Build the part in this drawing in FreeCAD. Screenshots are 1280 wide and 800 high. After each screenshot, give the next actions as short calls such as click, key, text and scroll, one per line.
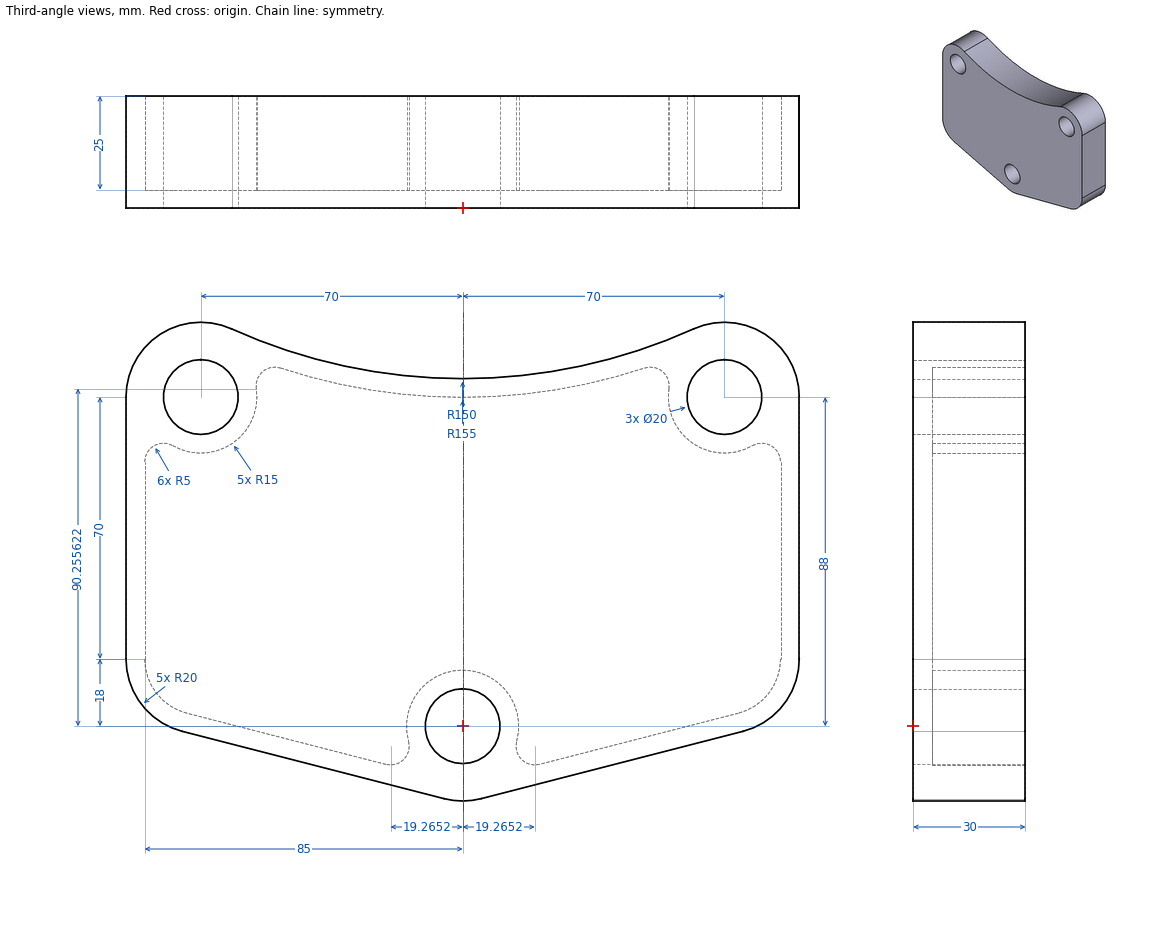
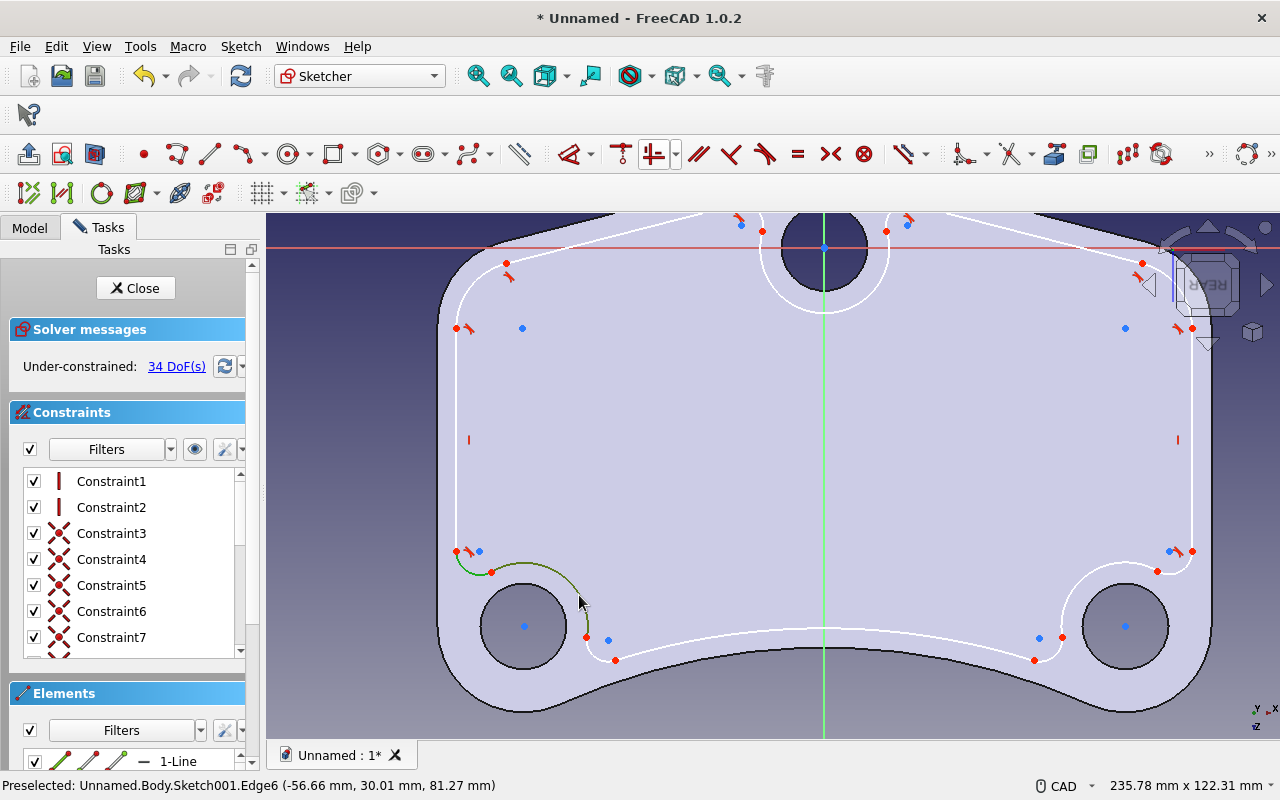
click(765, 154)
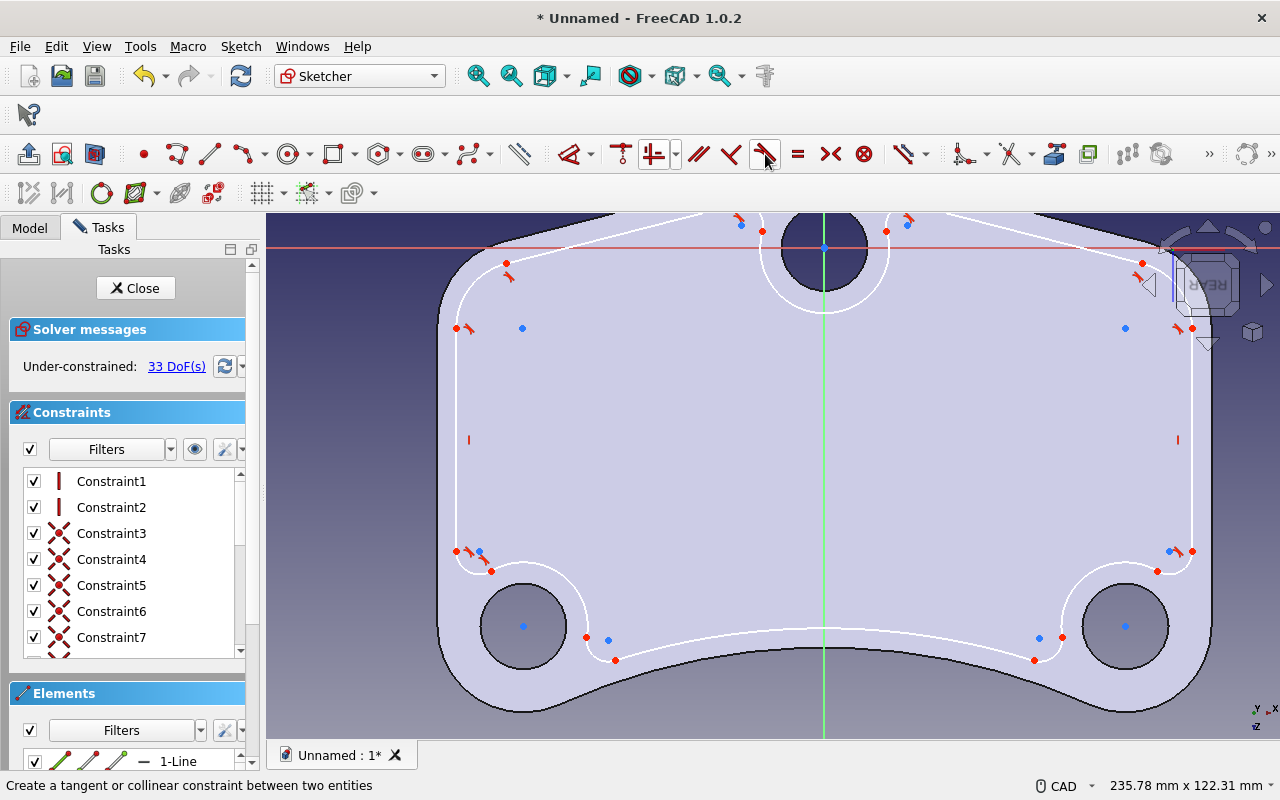
click(579, 595)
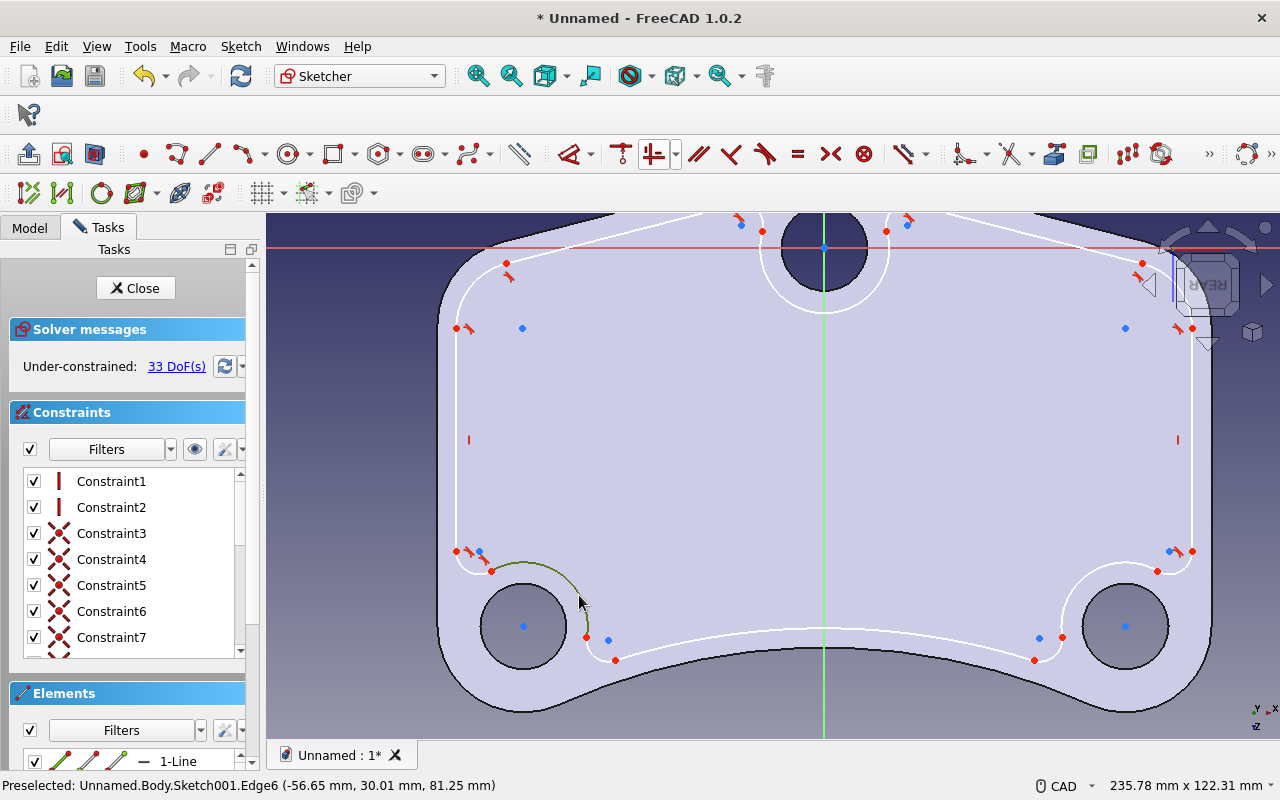
click(589, 650)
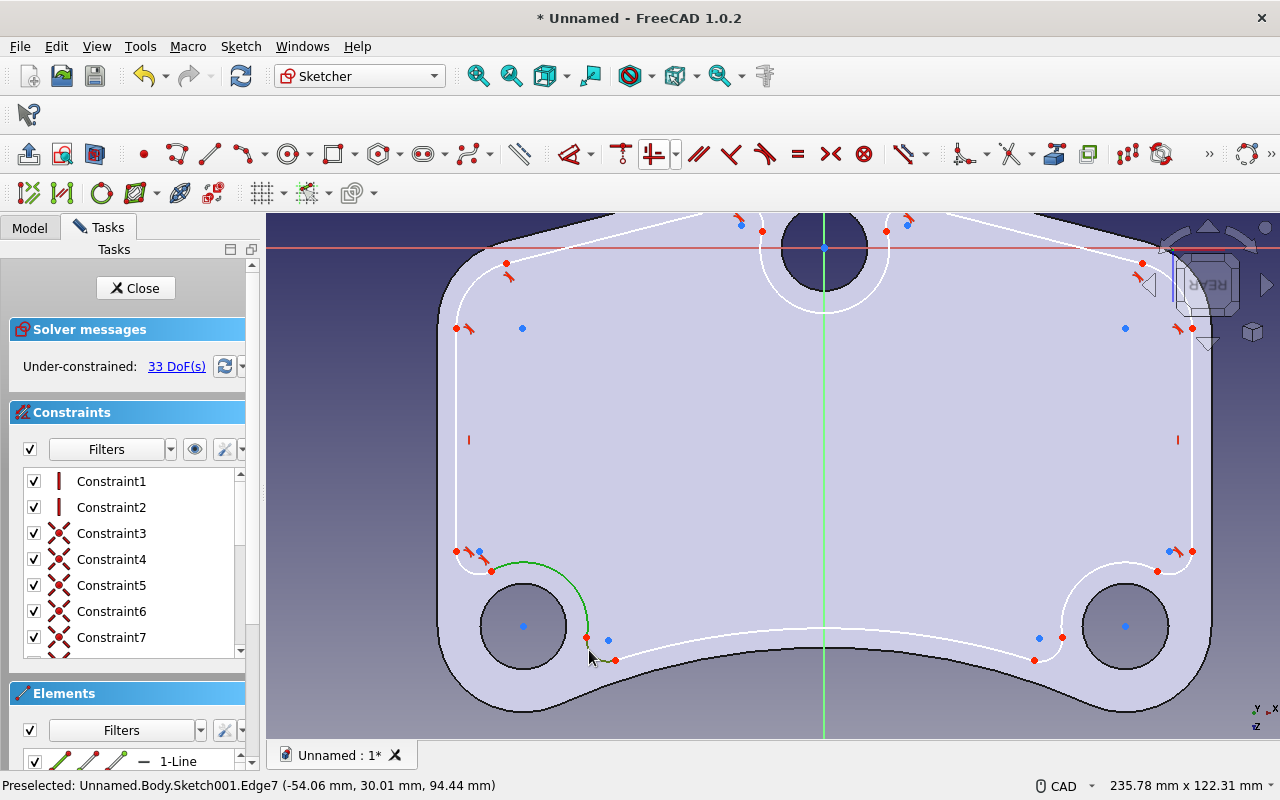
click(765, 154)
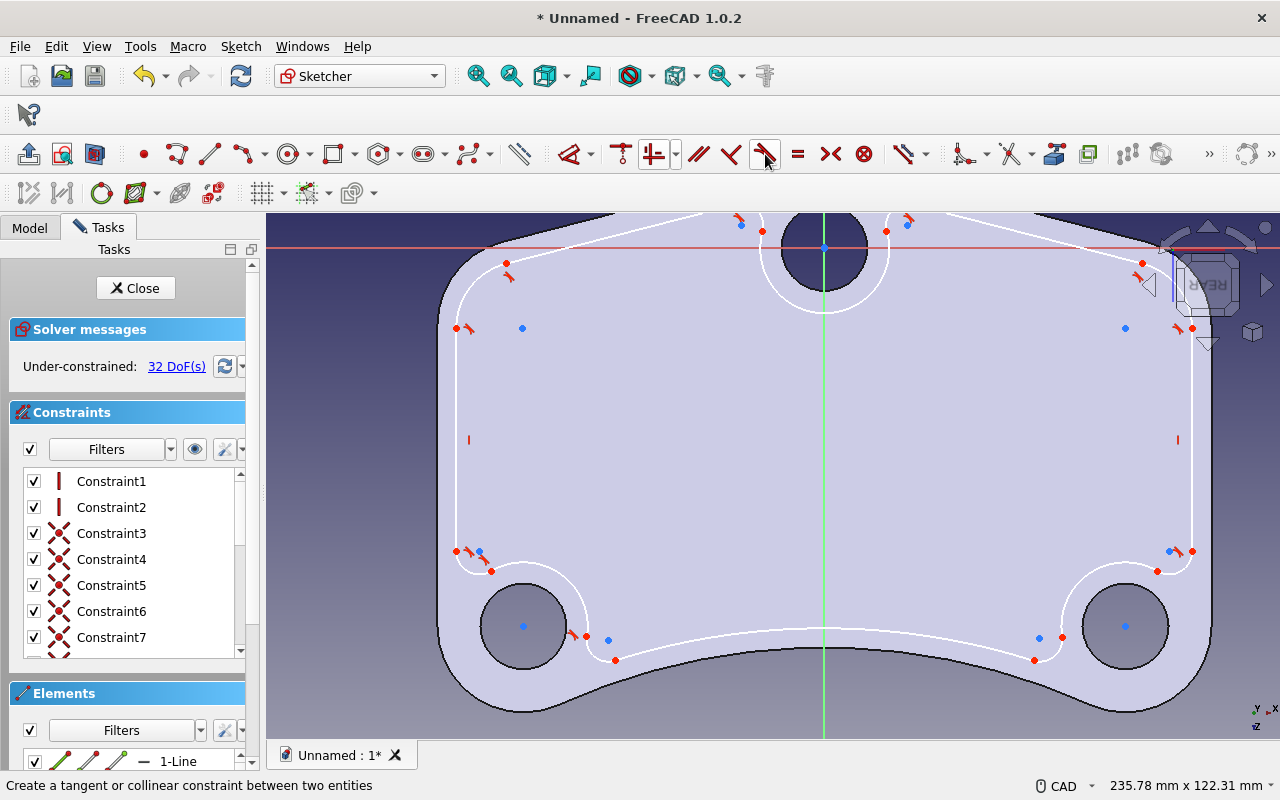
click(589, 650)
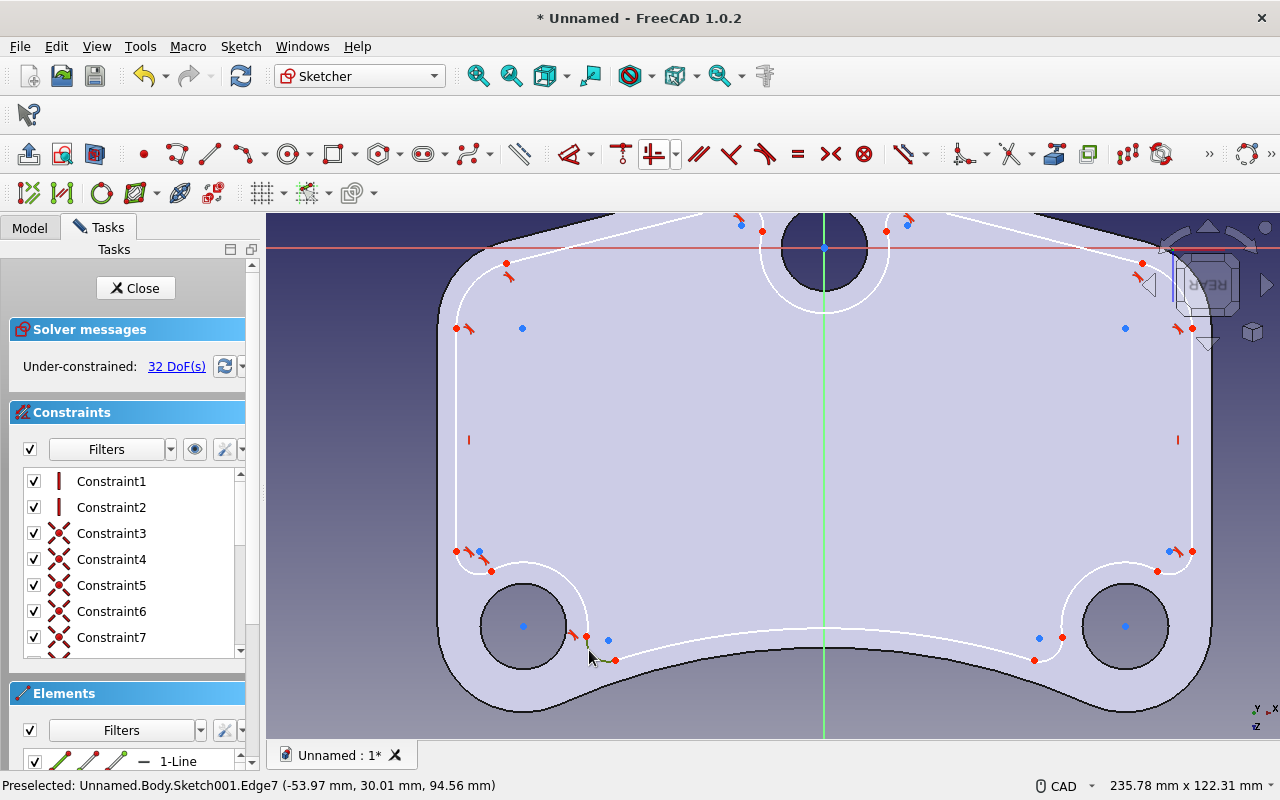
click(909, 634)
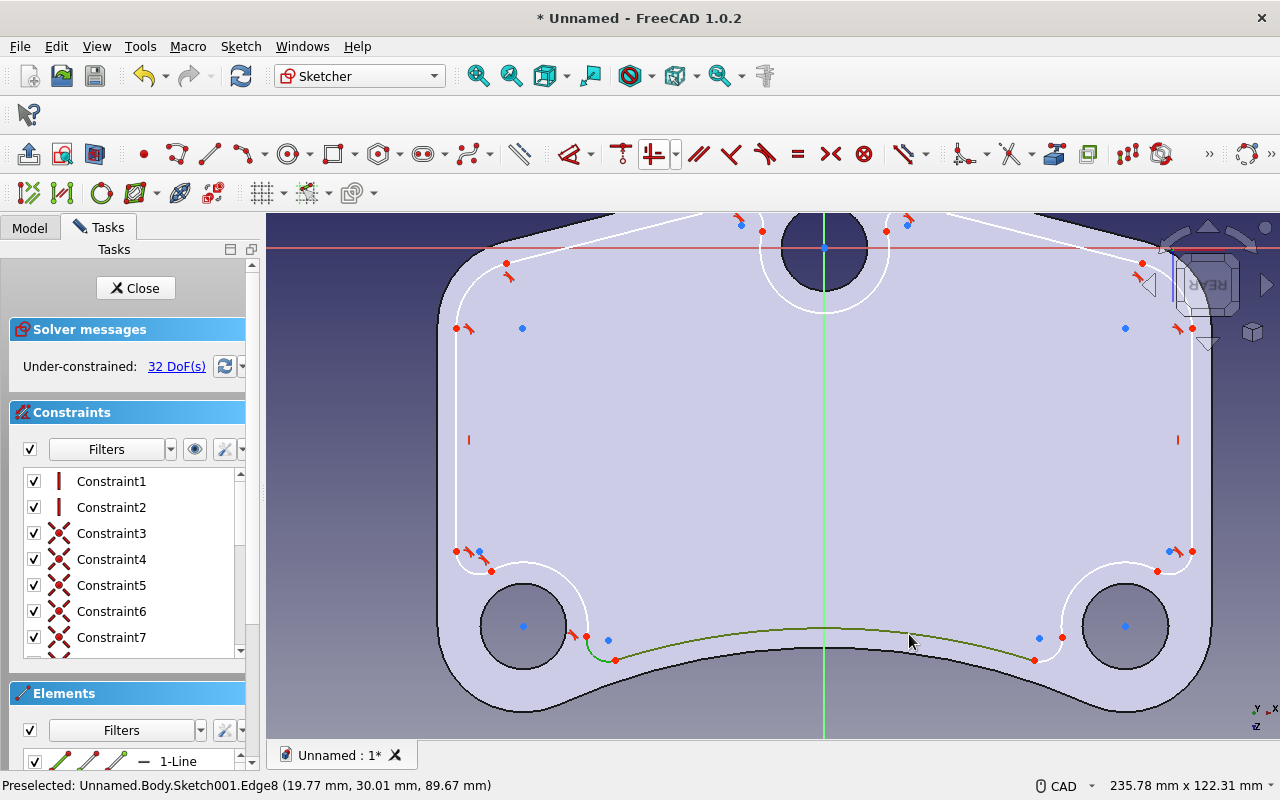
click(765, 154)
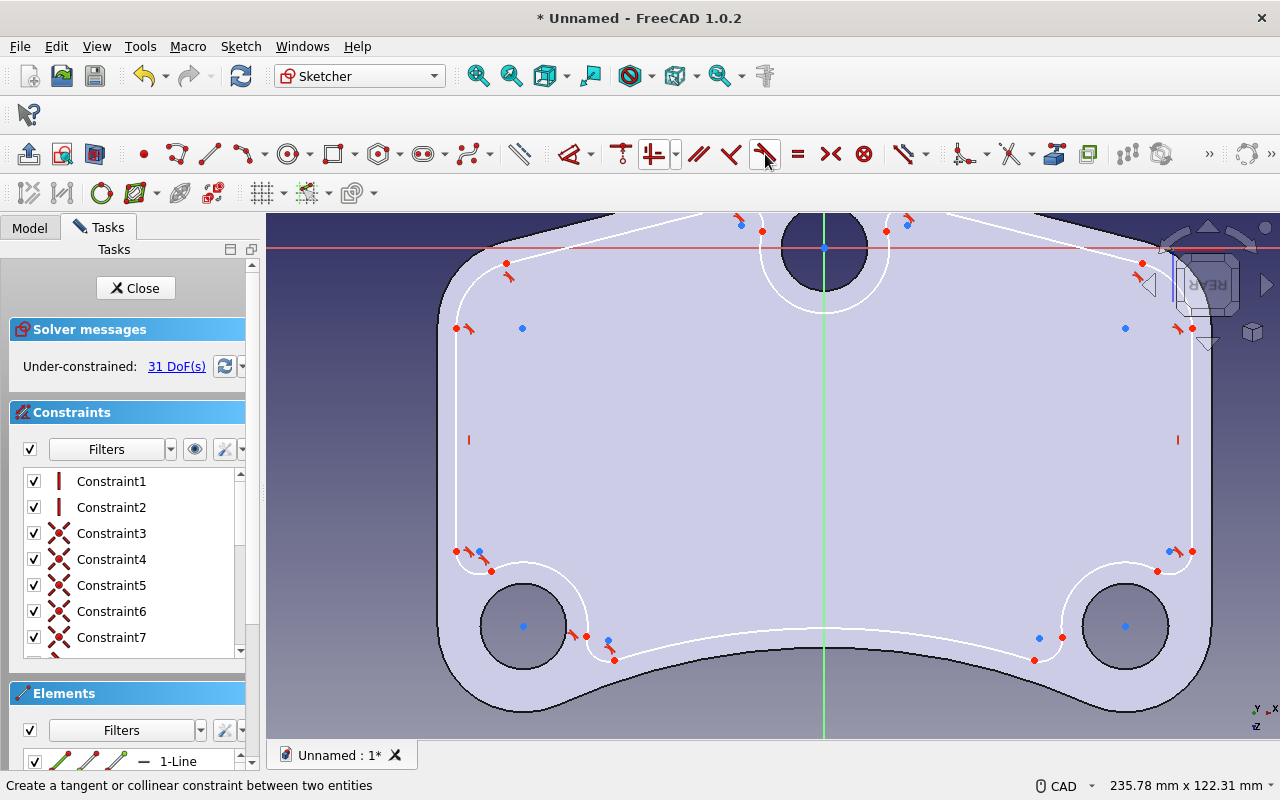
click(909, 634)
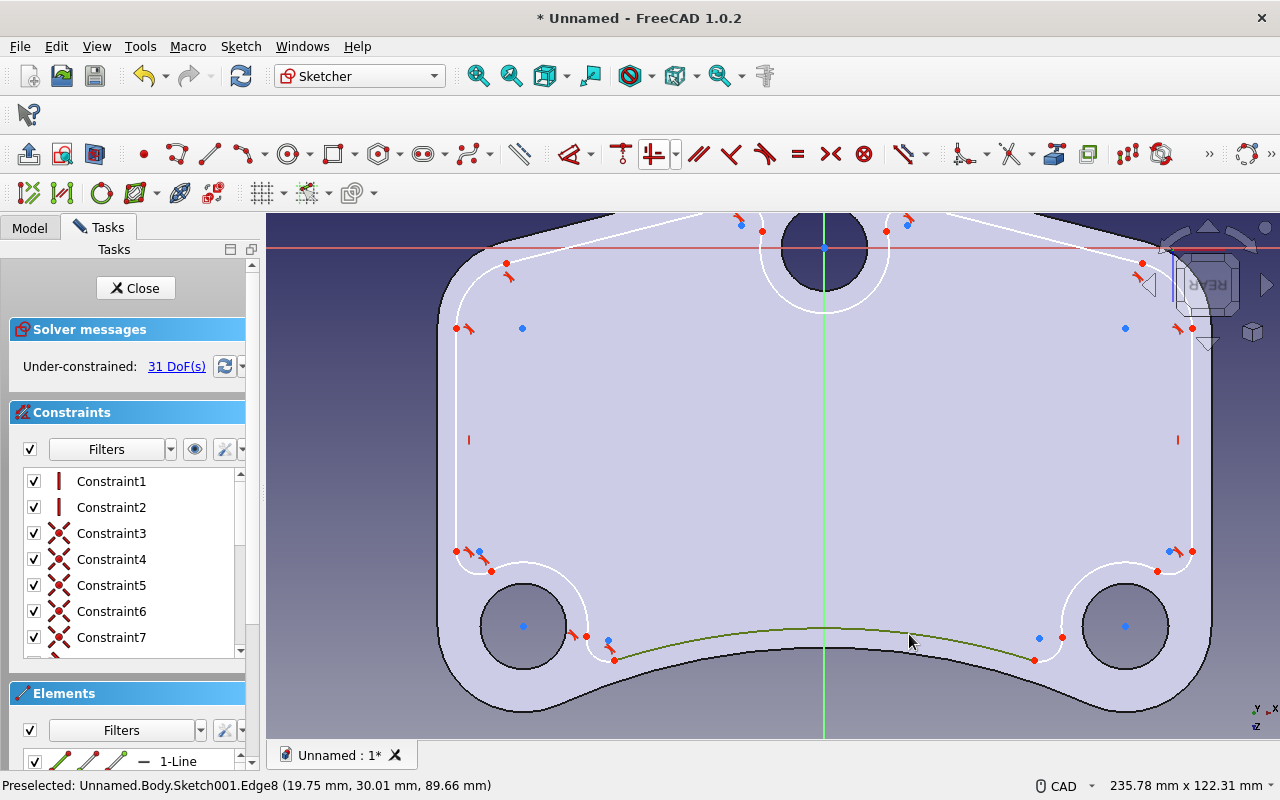
click(1047, 660)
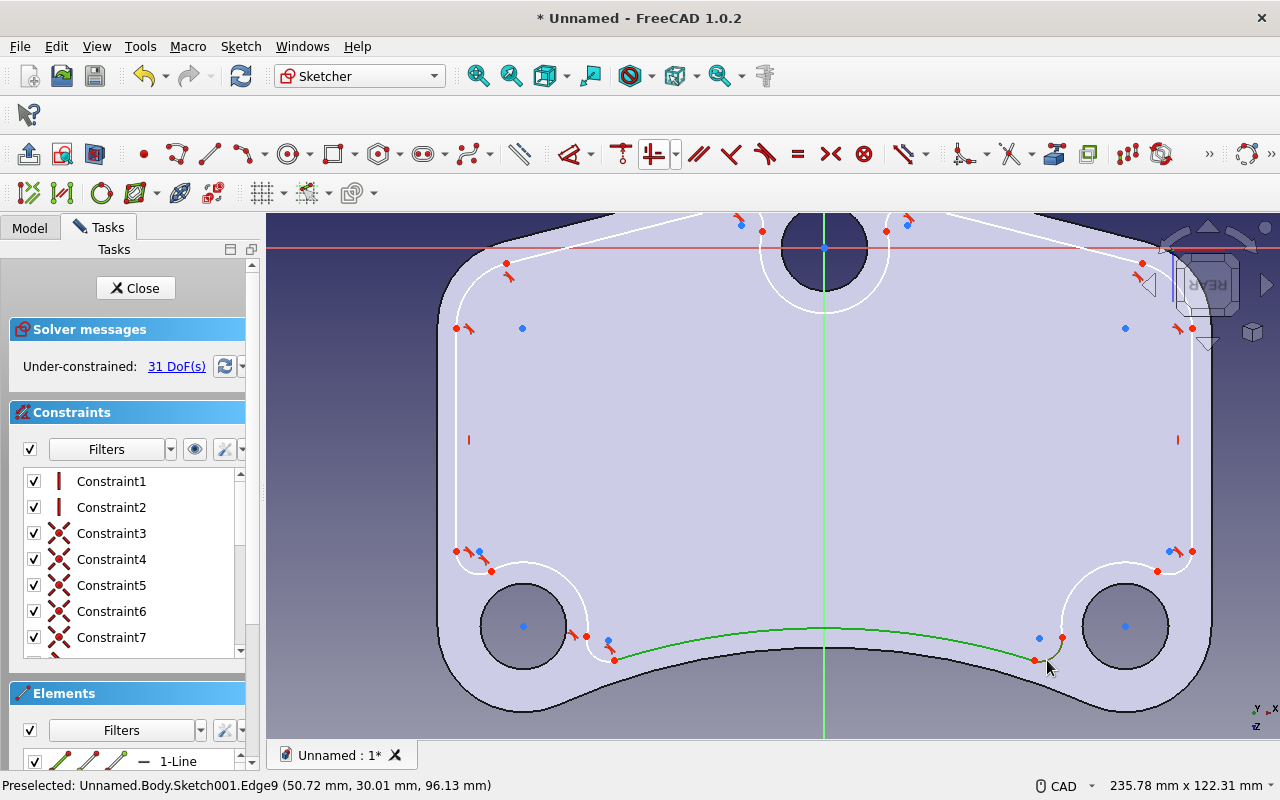
click(765, 154)